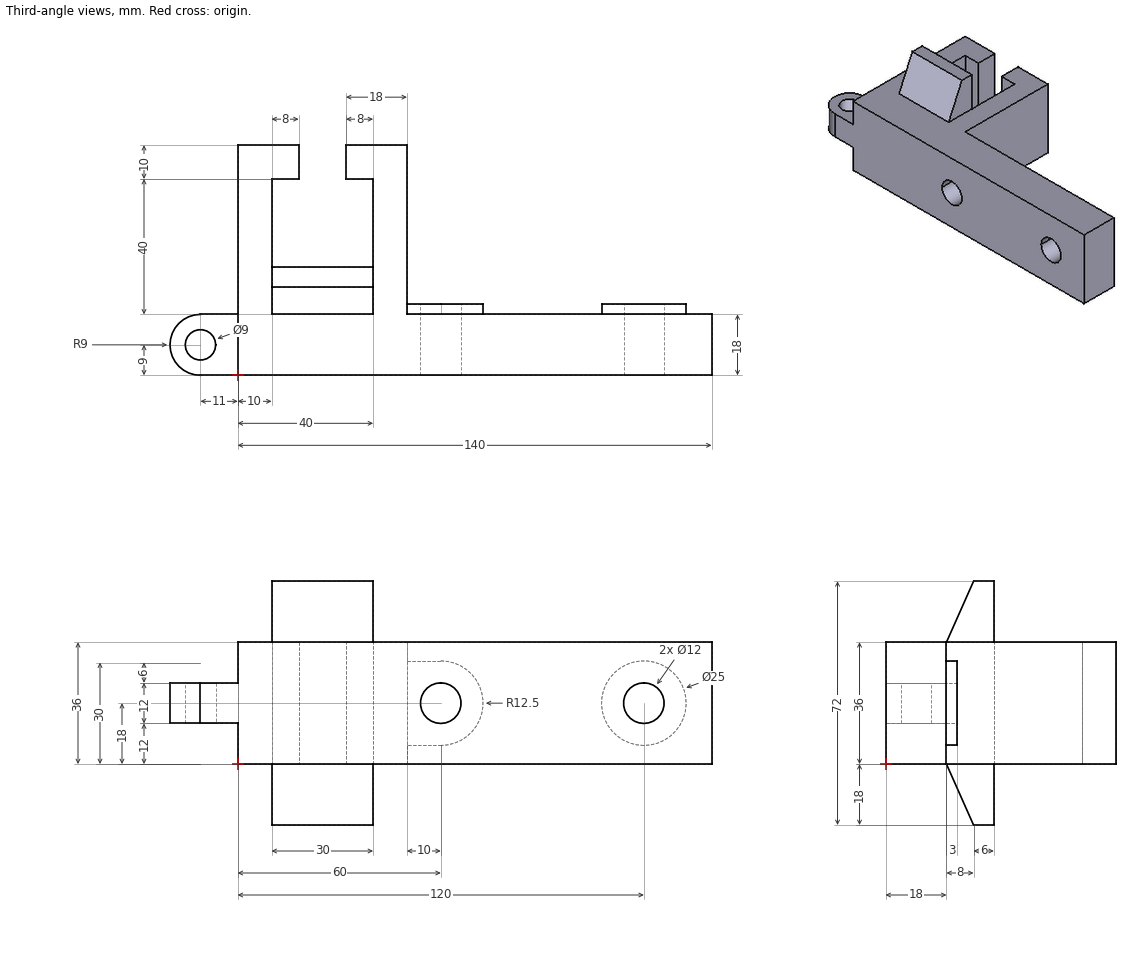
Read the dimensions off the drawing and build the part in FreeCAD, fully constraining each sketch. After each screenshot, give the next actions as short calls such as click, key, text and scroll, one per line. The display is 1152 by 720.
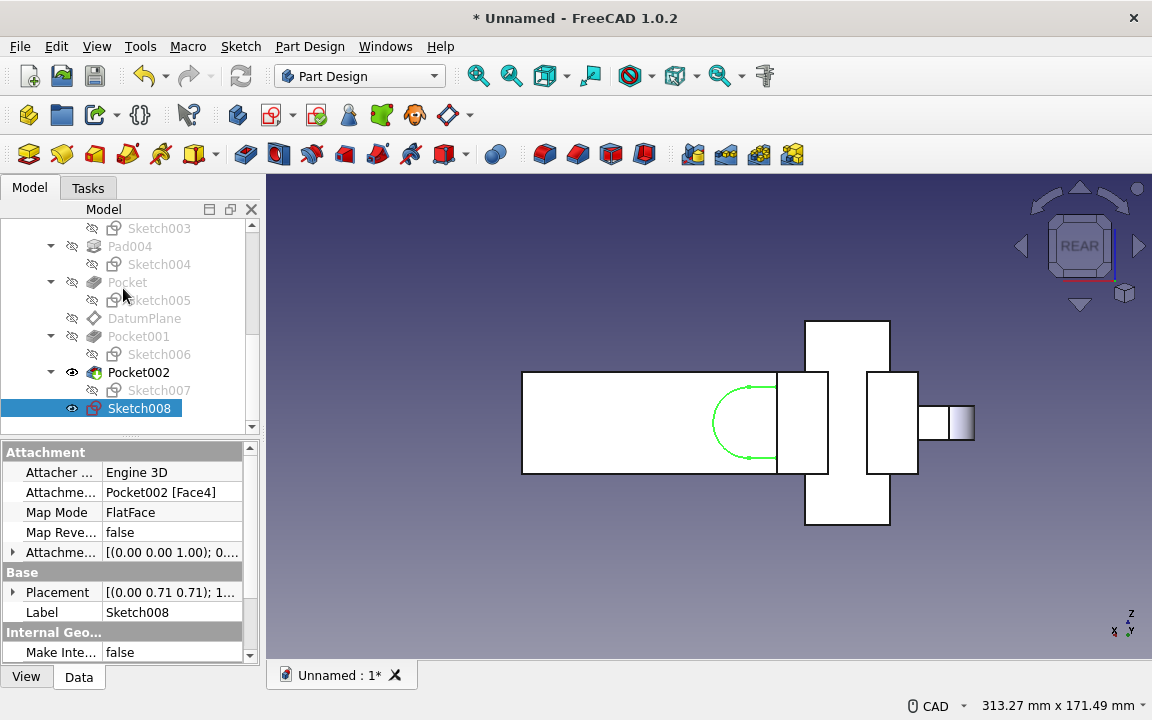
click(29, 154)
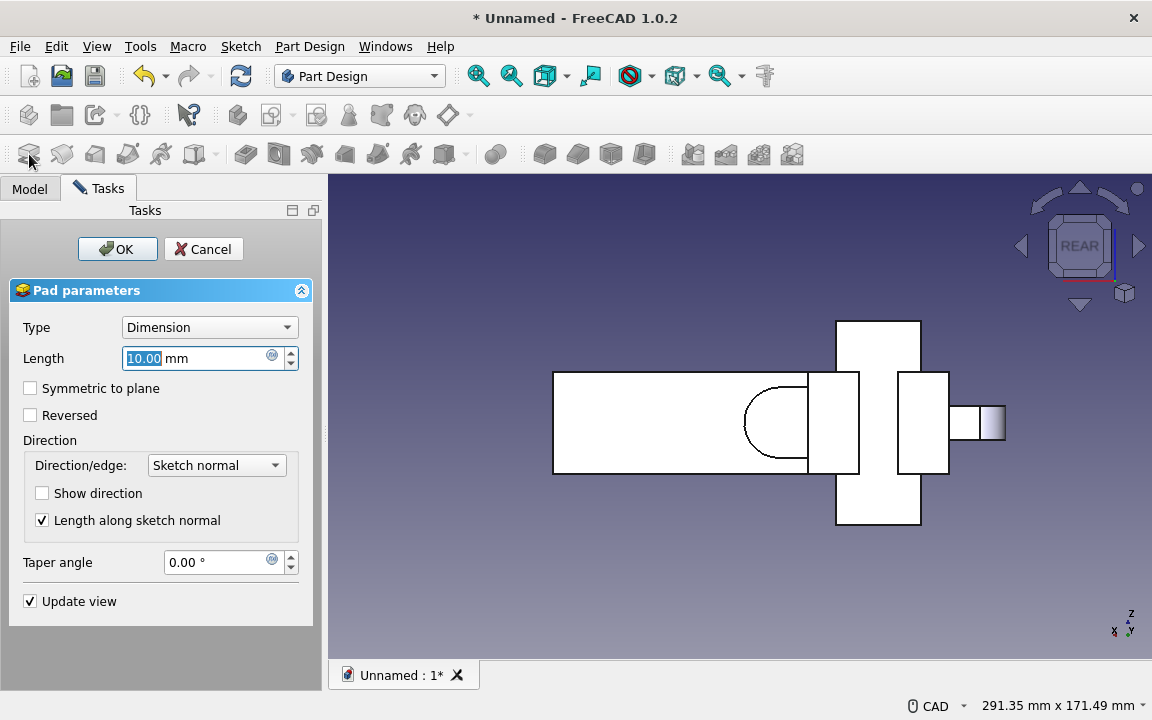
text(3)
key(Tab)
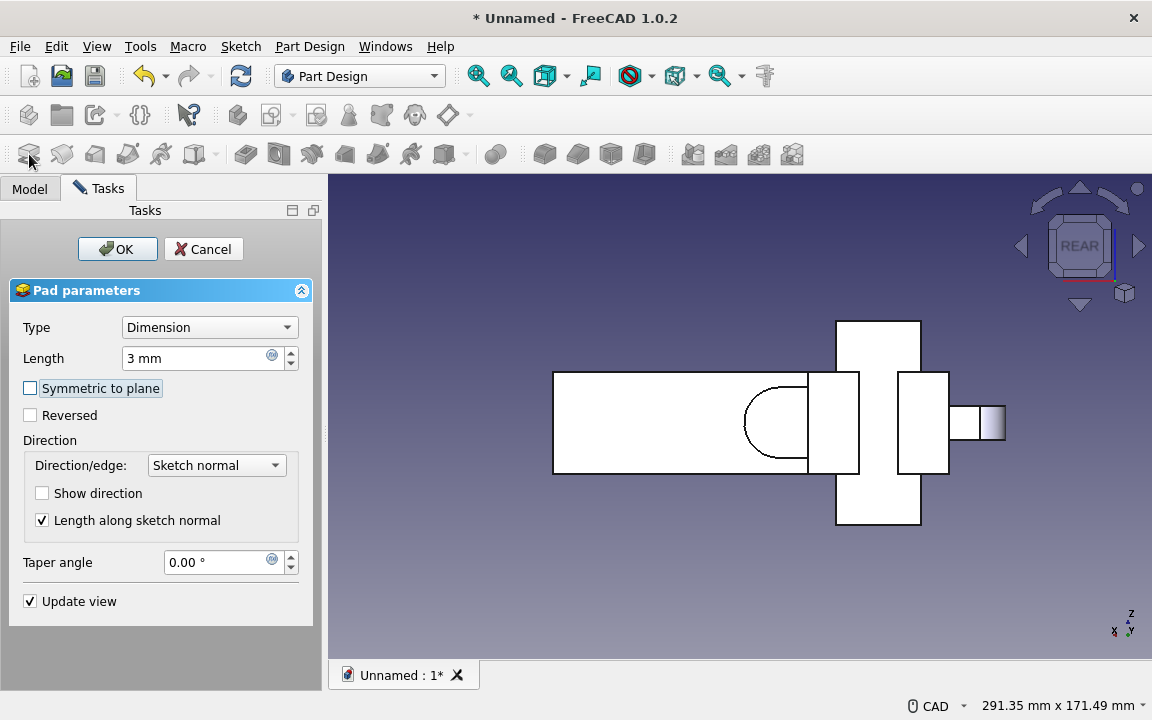
click(118, 249)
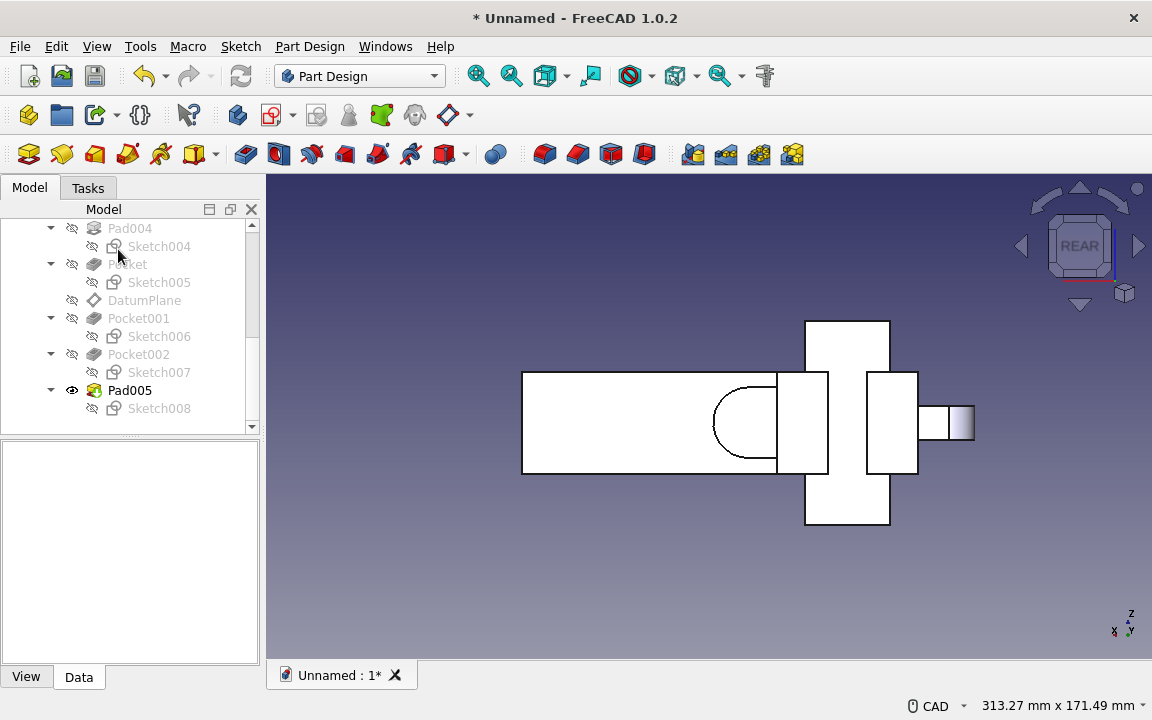
click(577, 422)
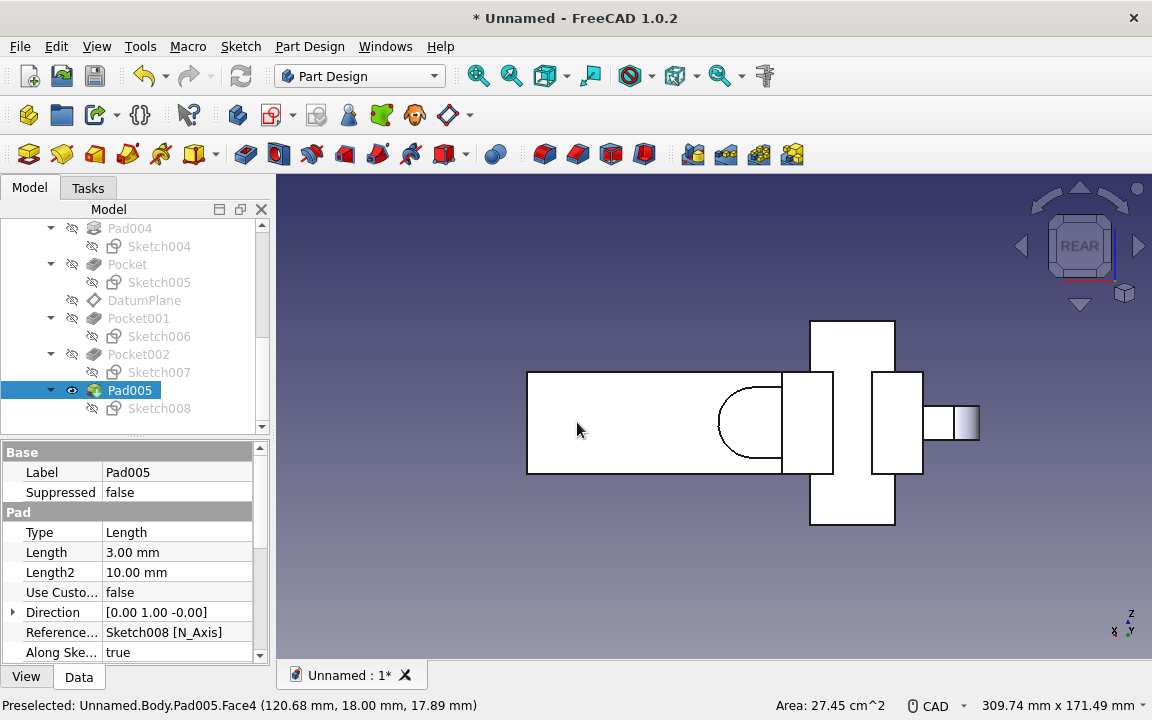
click(270, 116)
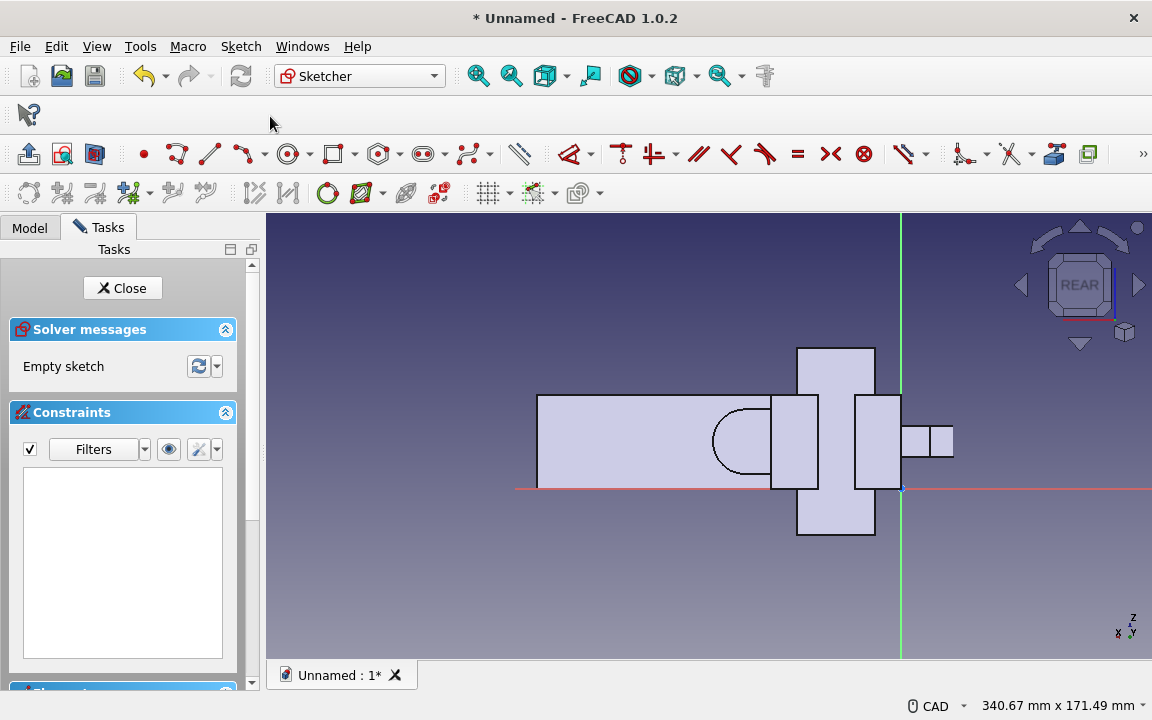
click(95, 154)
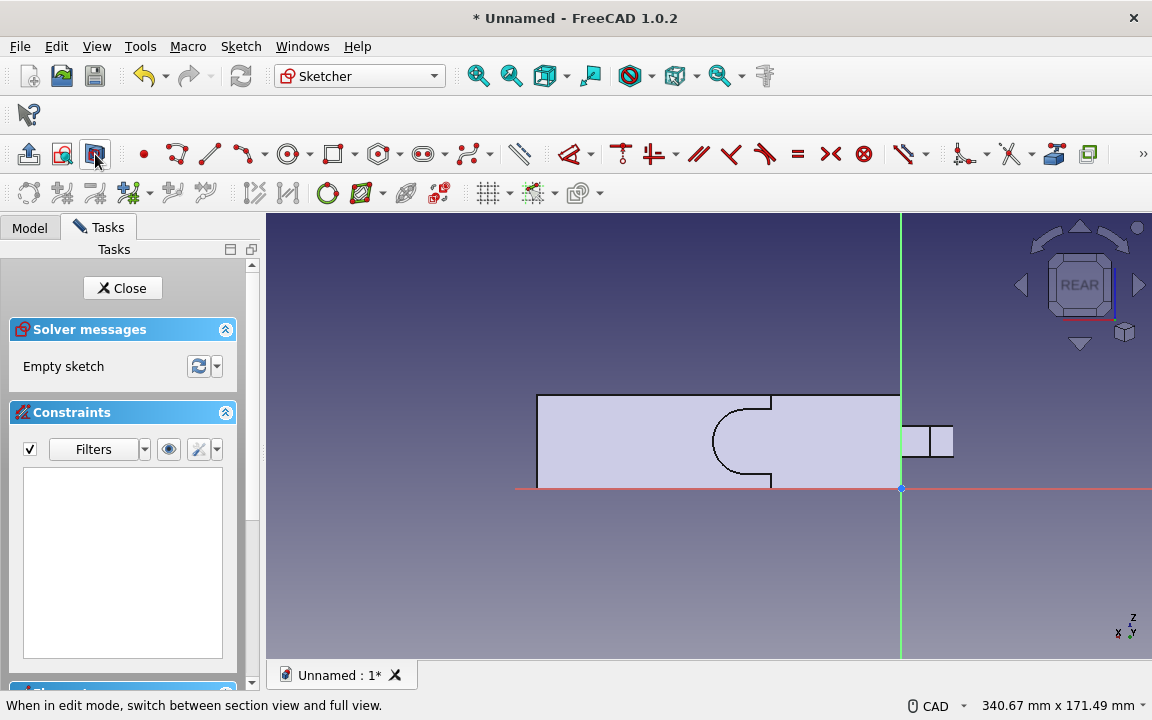
scroll(573, 444, up, 7)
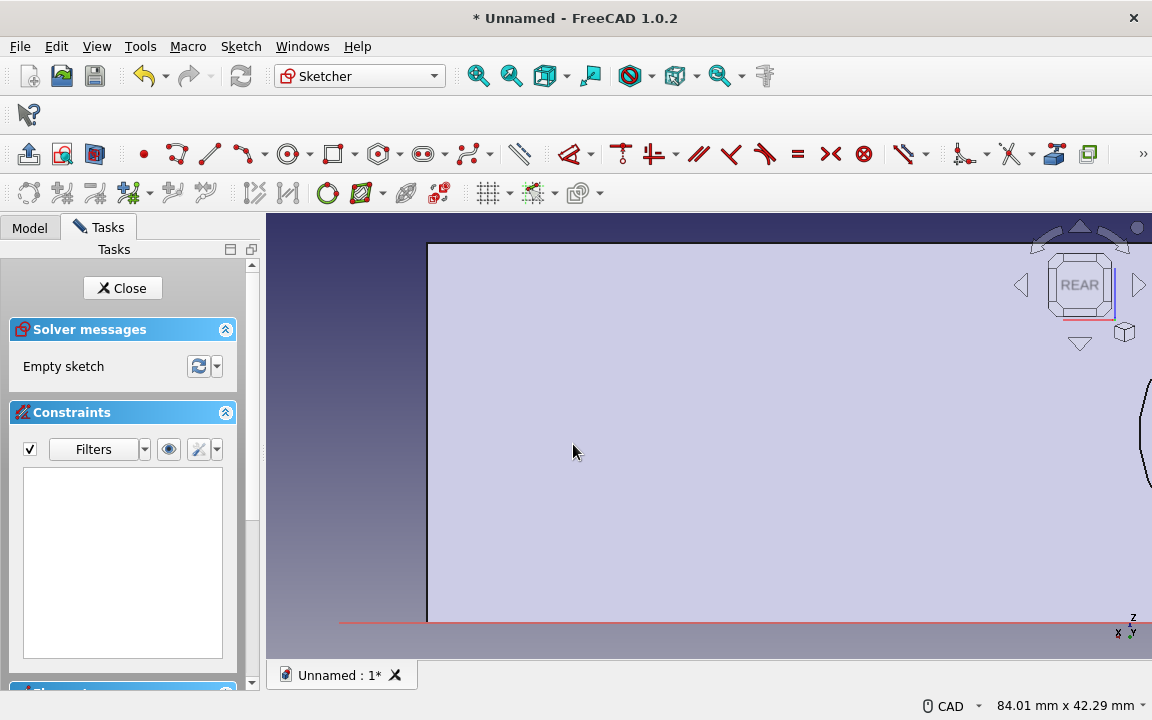
key(g)
key(c)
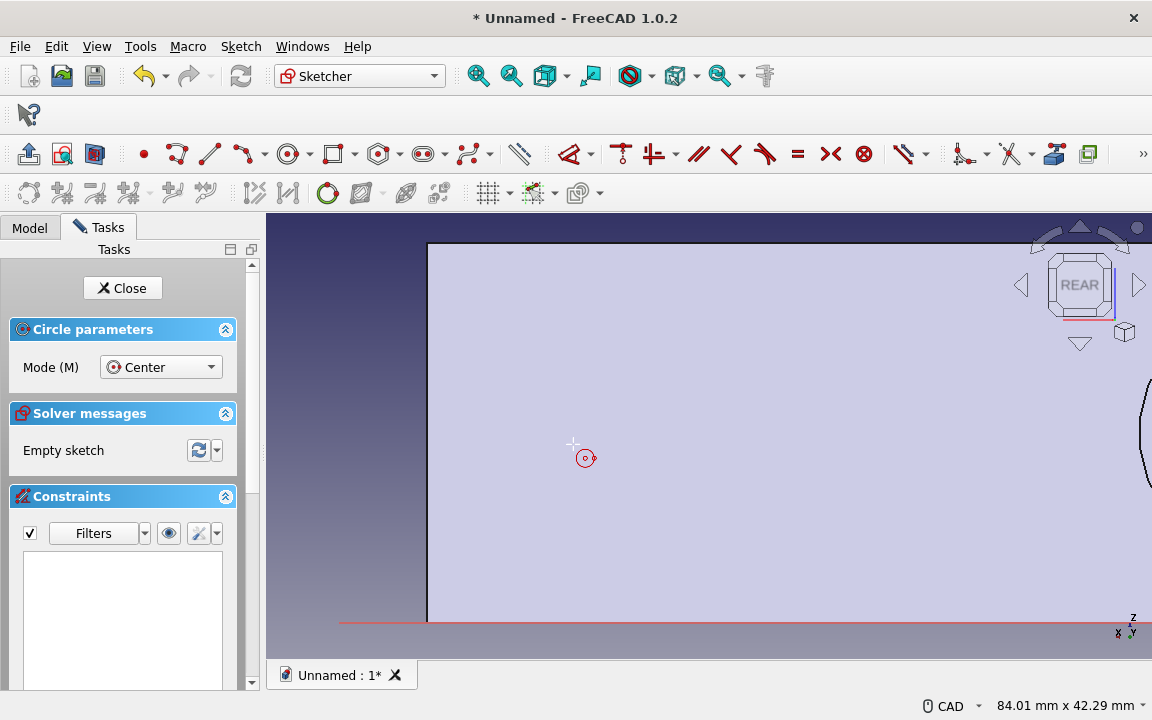
click(638, 433)
click(732, 340)
key(Escape)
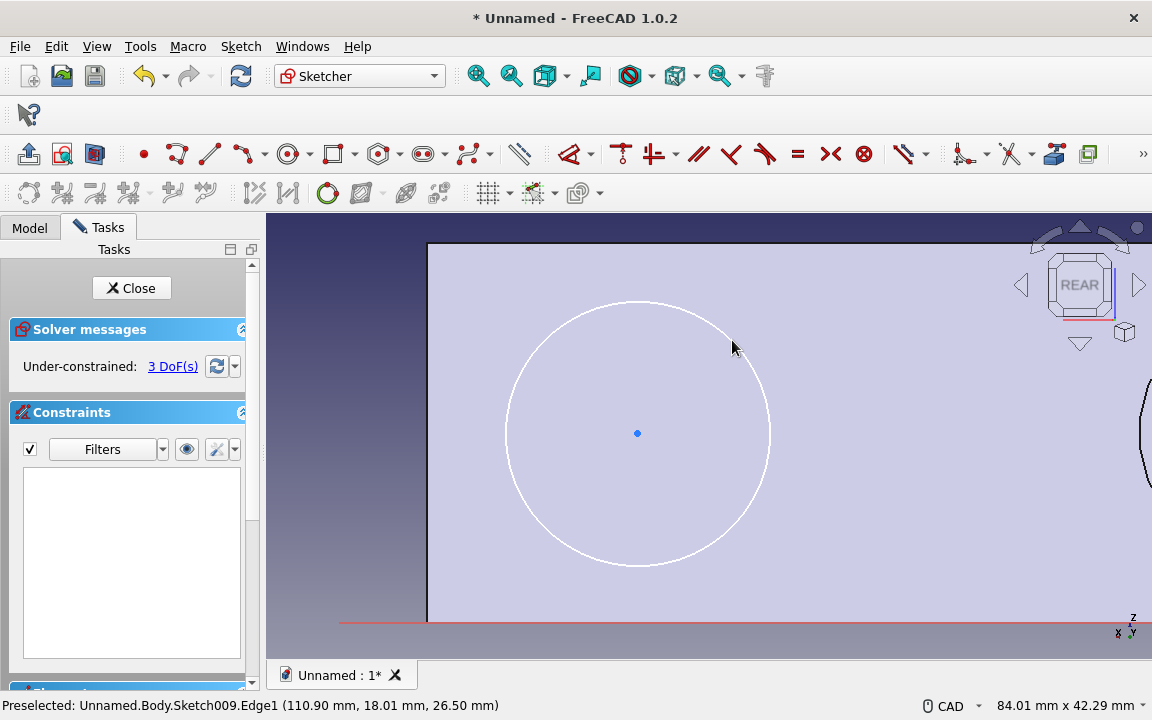
click(568, 154)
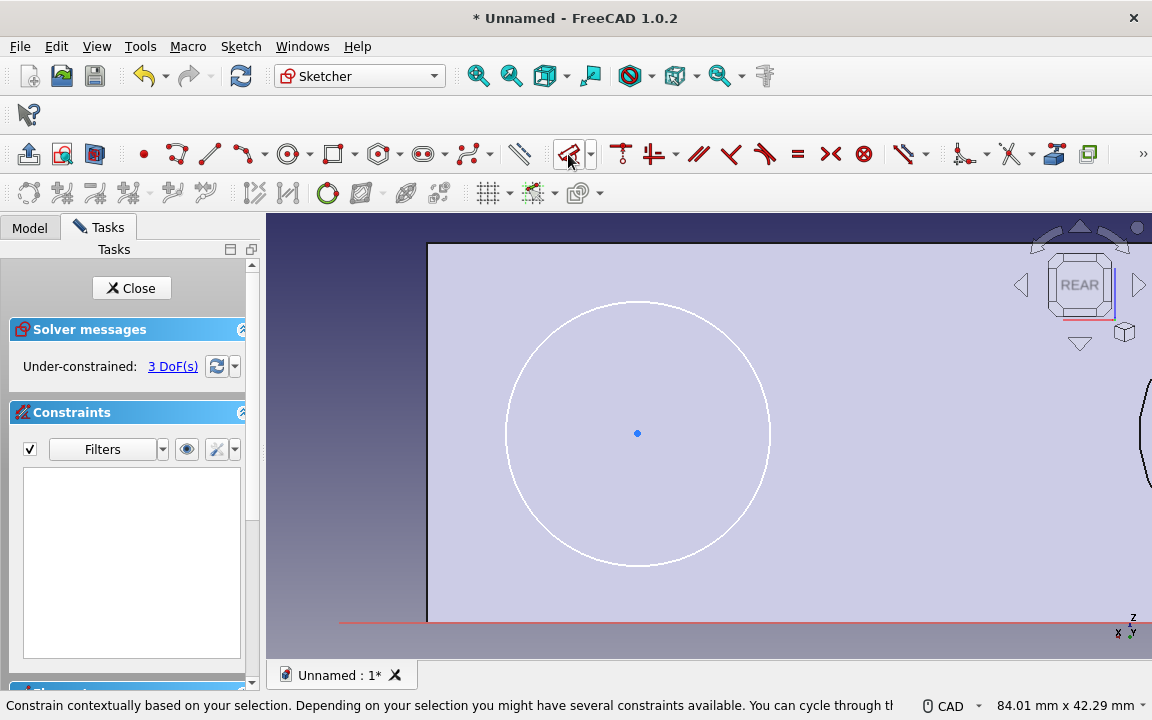
click(731, 340)
click(754, 317)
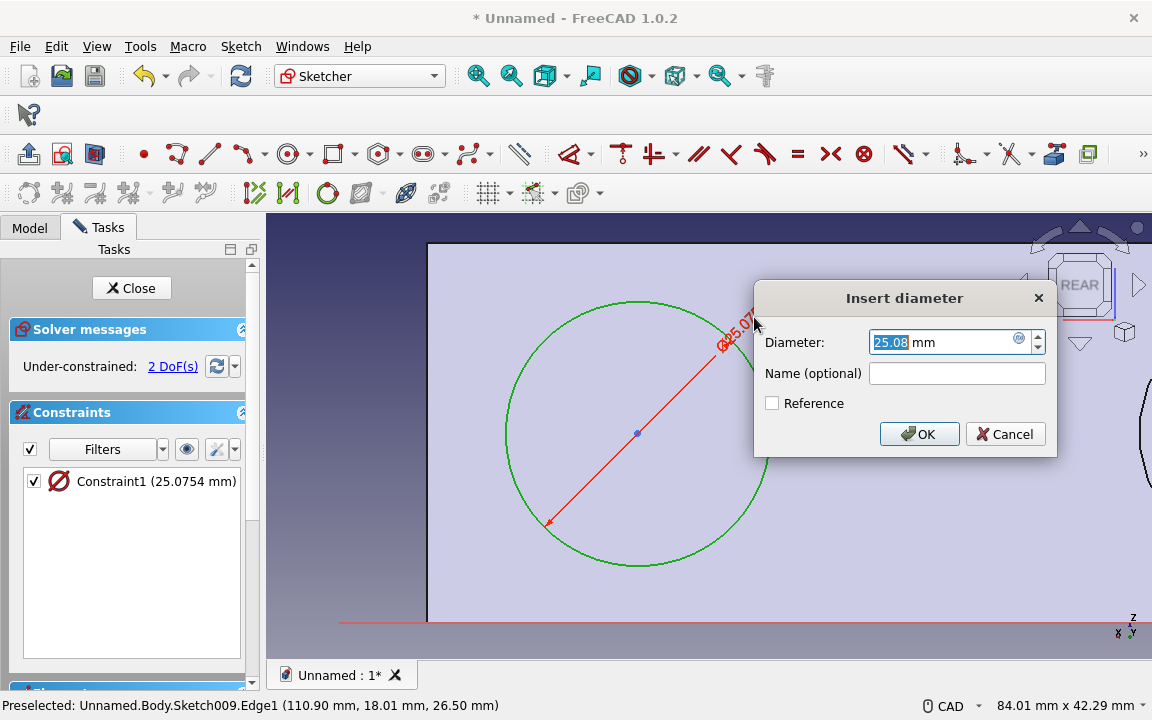
text(25)
key(Return)